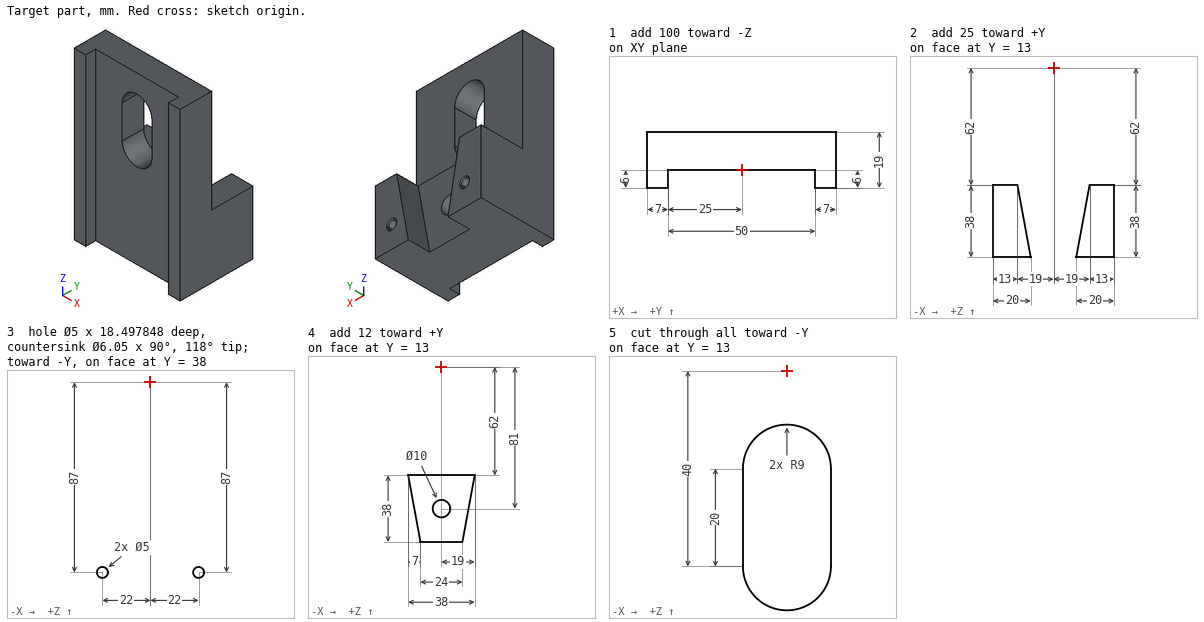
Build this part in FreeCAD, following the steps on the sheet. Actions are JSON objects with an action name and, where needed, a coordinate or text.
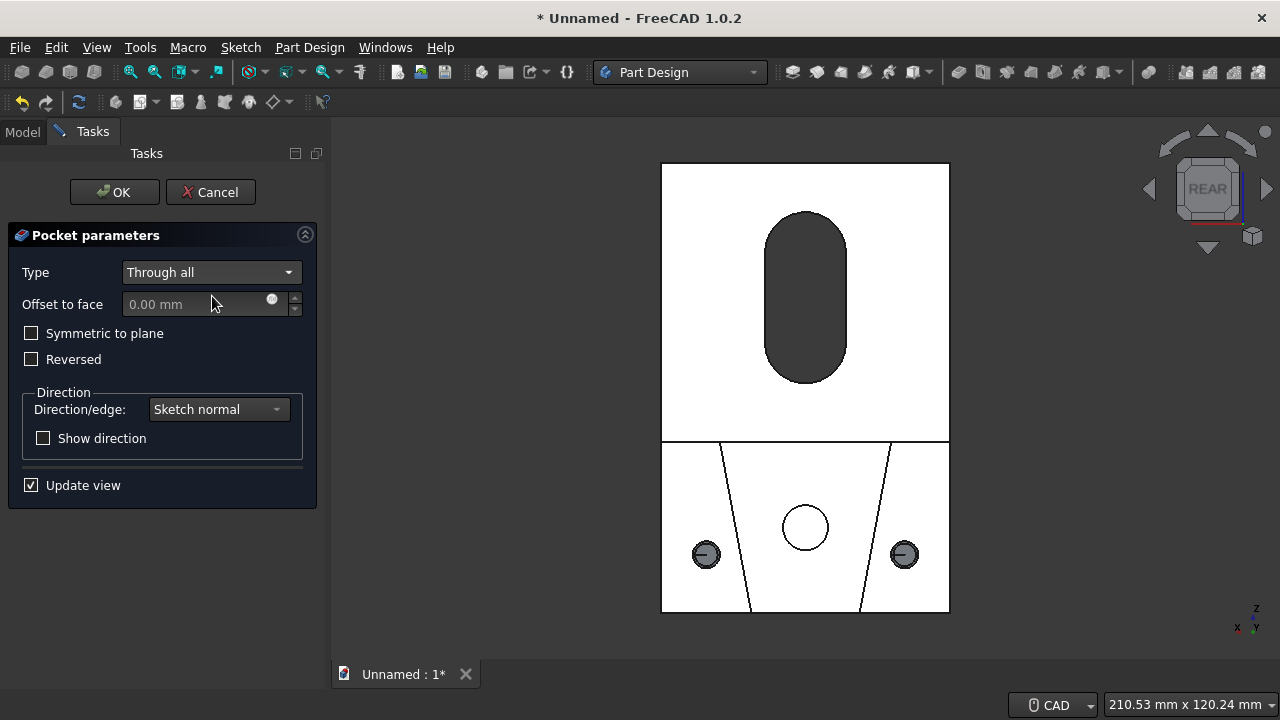
{"action": "left_click", "coordinate": [115, 192]}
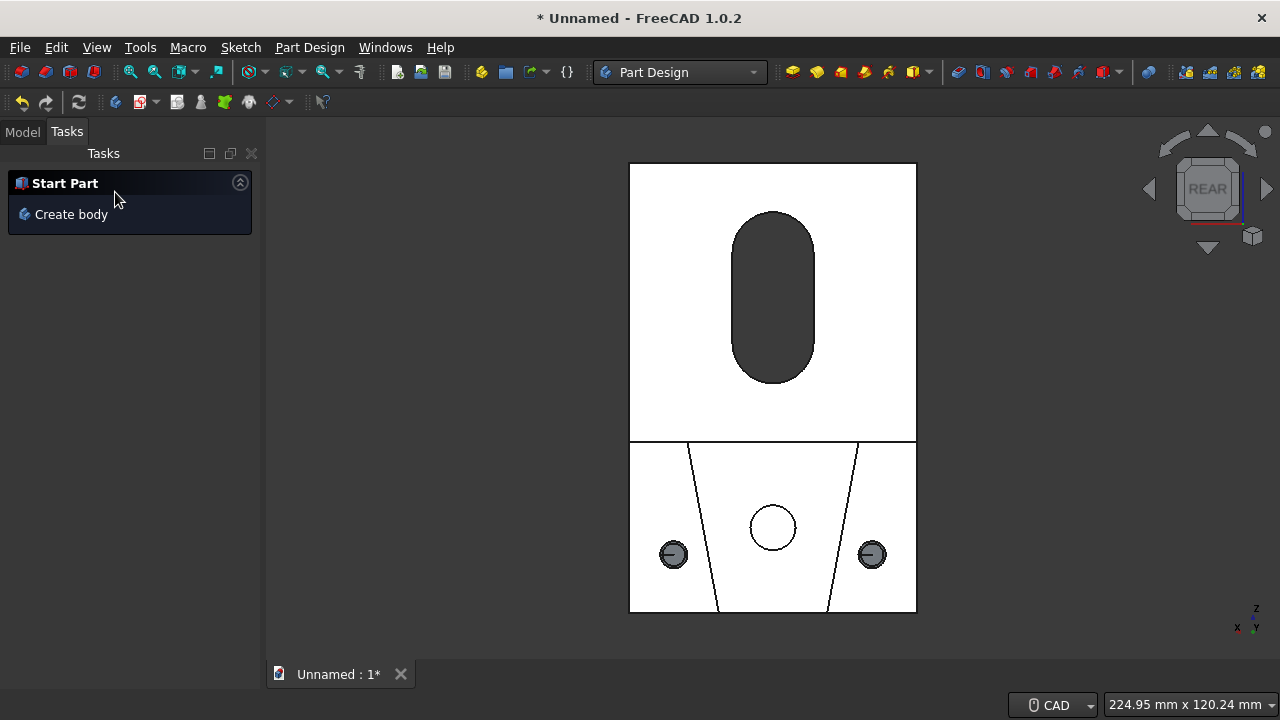
{"action": "key", "text": "0"}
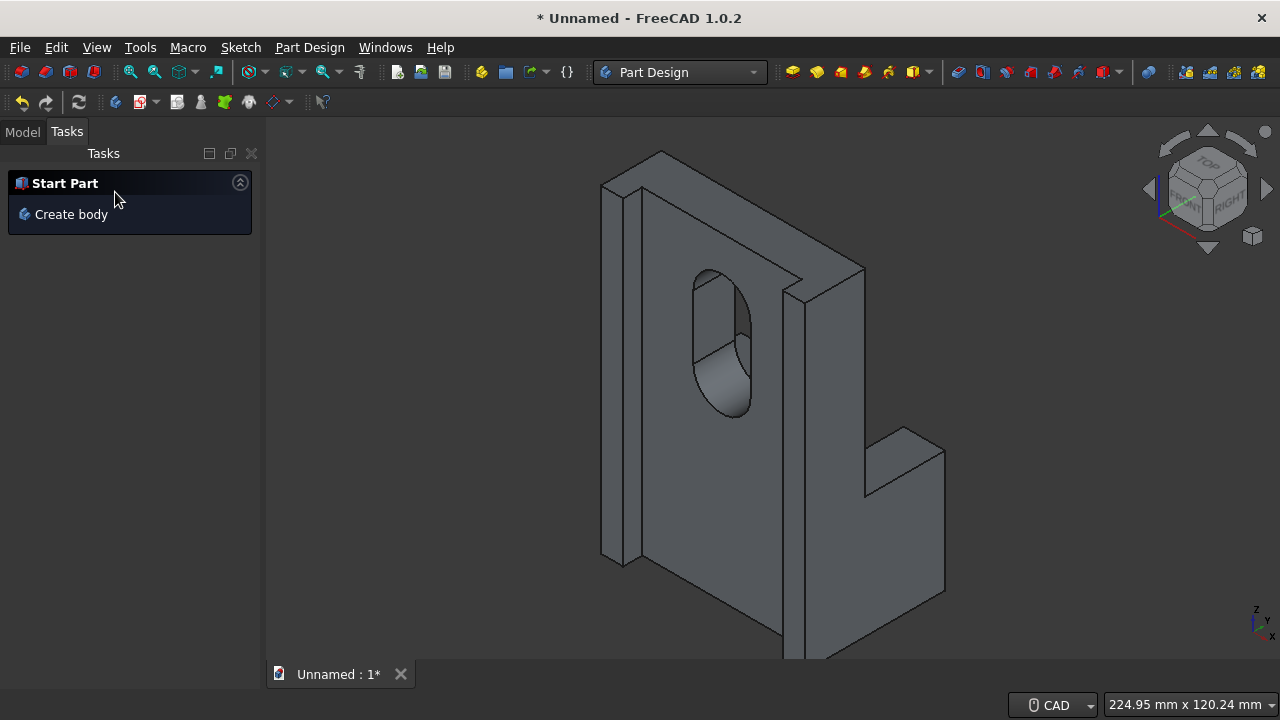
{"action": "key", "text": "v f"}